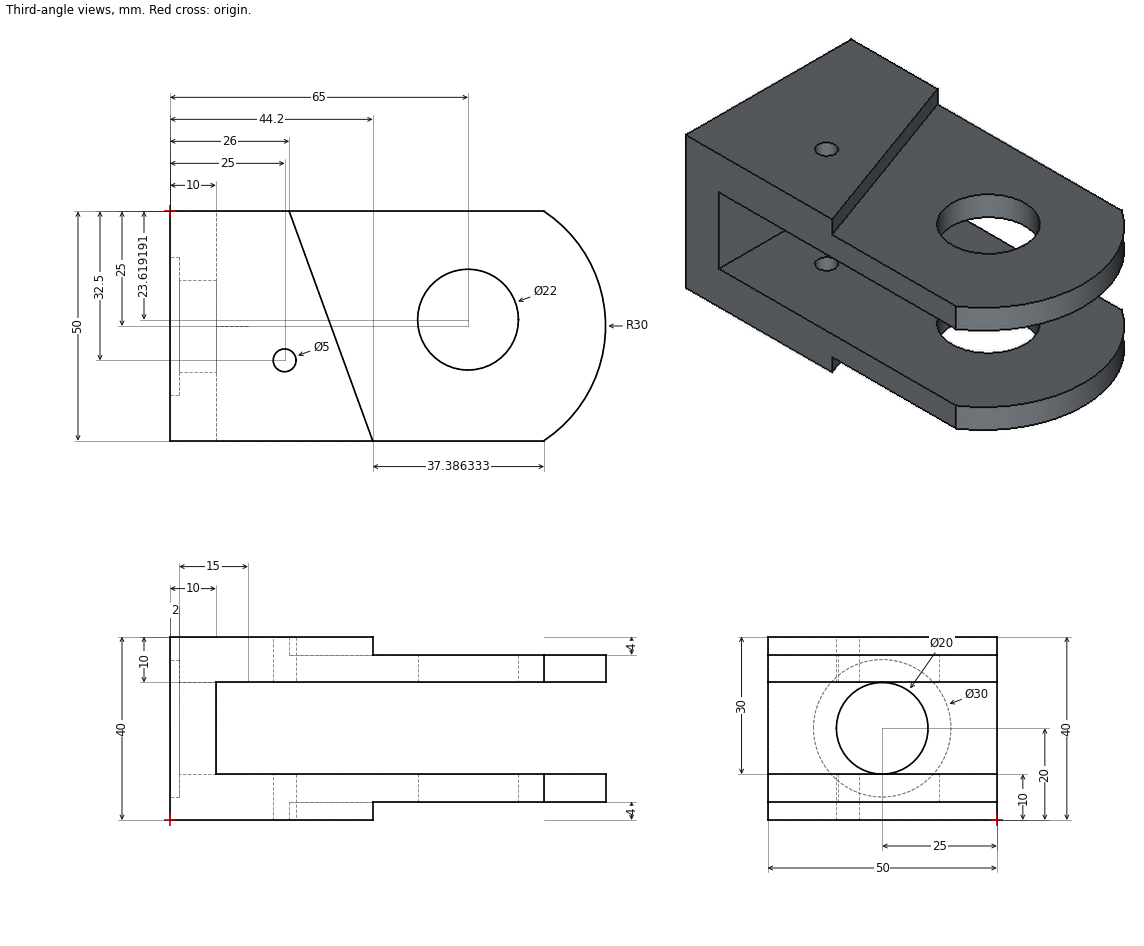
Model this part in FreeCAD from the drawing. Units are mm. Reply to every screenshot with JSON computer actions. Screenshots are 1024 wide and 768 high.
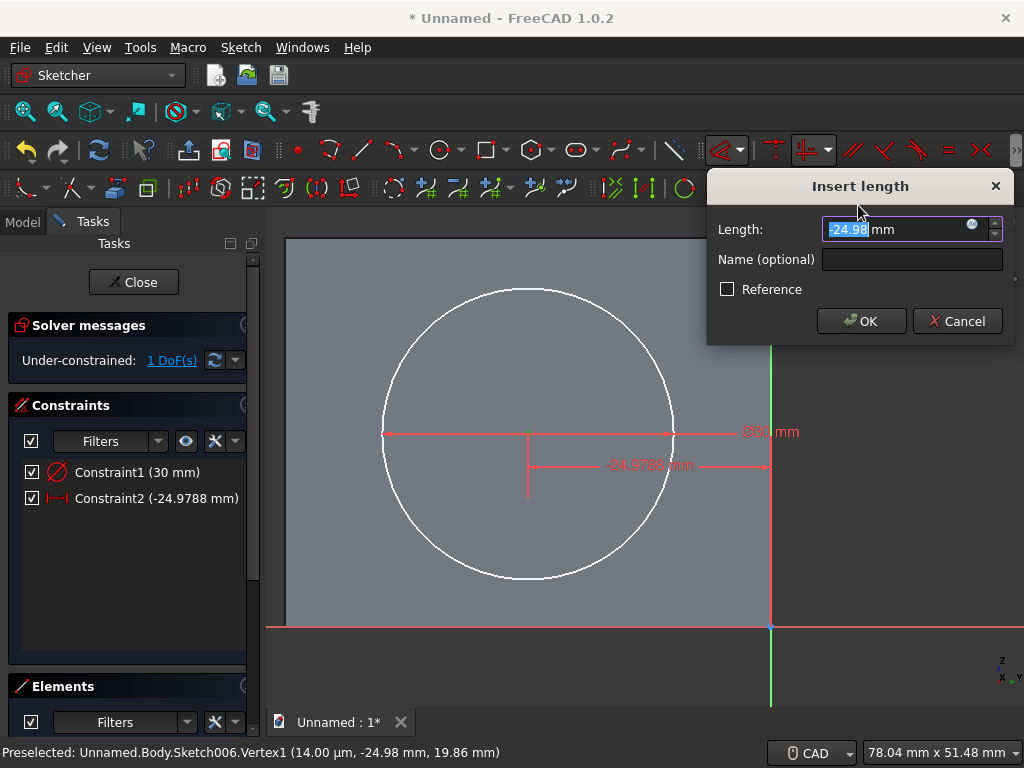
{"action": "type", "text": "-25"}
{"action": "key", "text": "Return"}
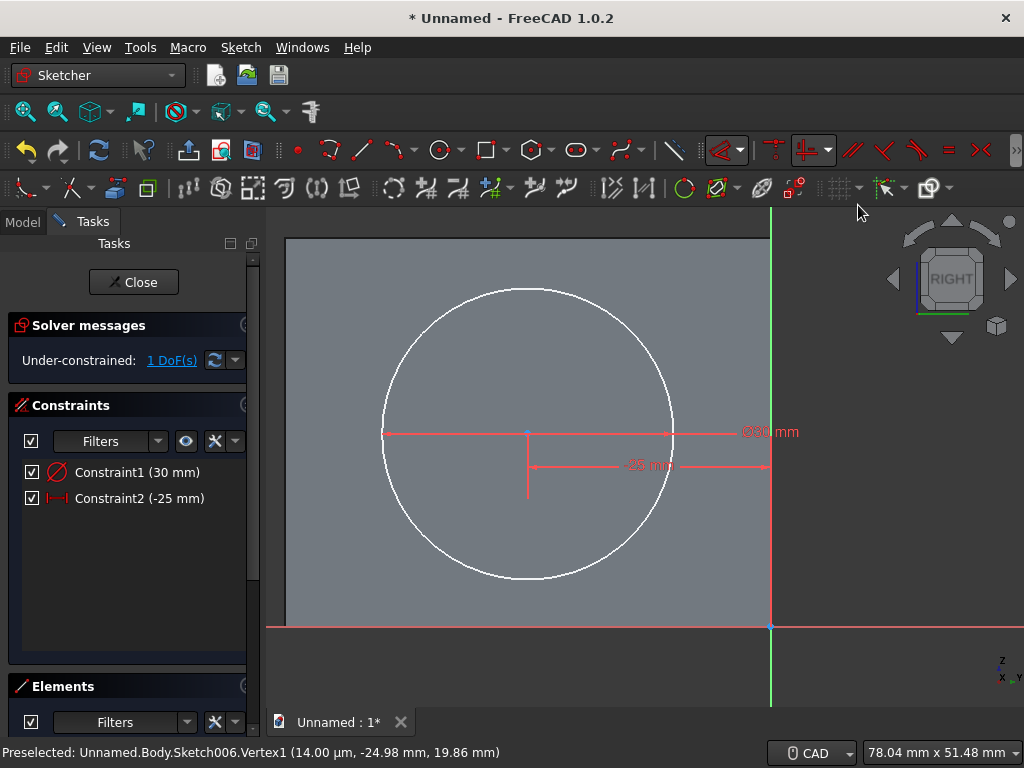
{"action": "left_click", "coordinate": [528, 434]}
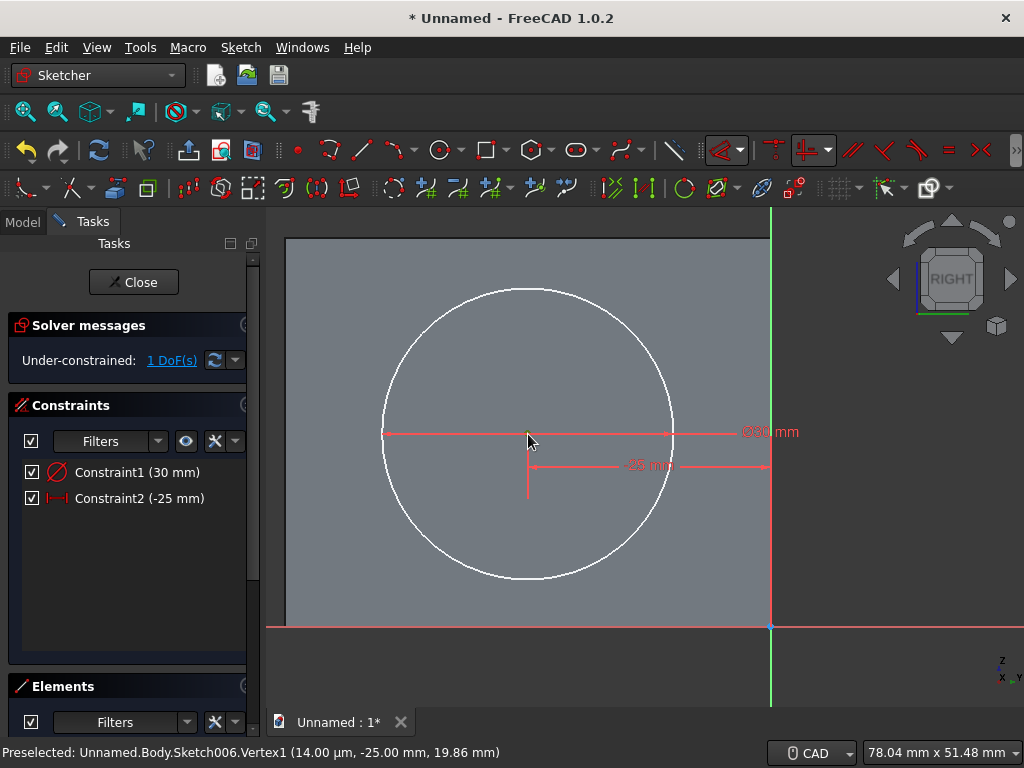
{"action": "key", "text": "i"}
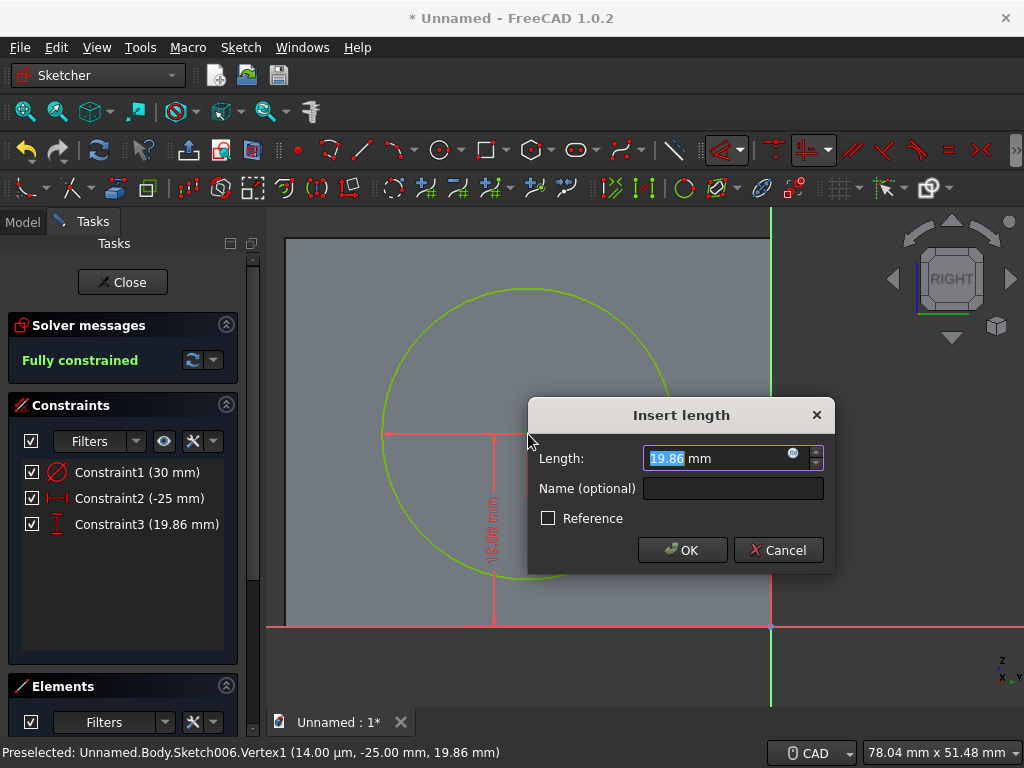
{"action": "type", "text": "20"}
{"action": "key", "text": "Return"}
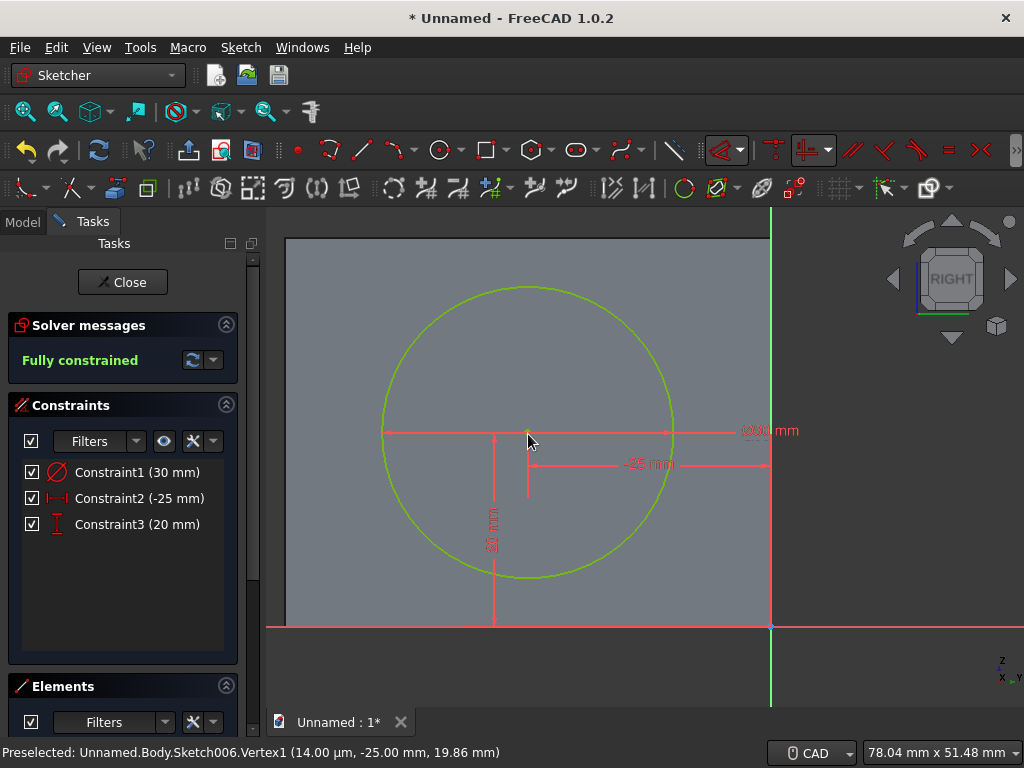
{"action": "left_click", "coordinate": [123, 282]}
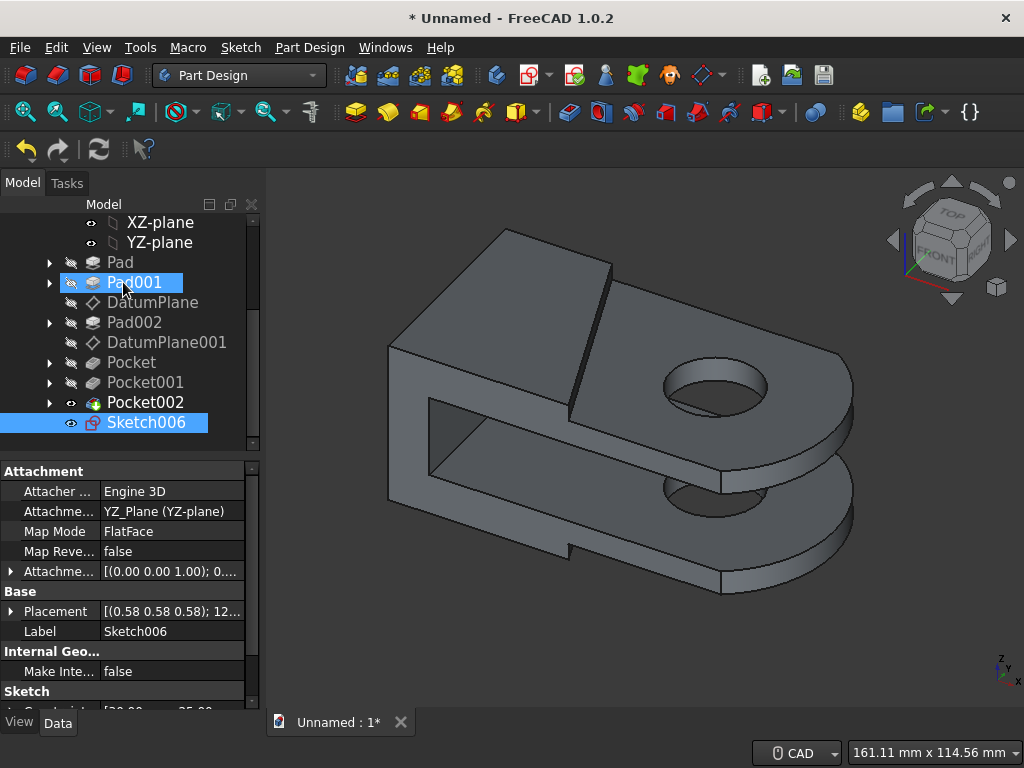
{"action": "left_click", "coordinate": [570, 112]}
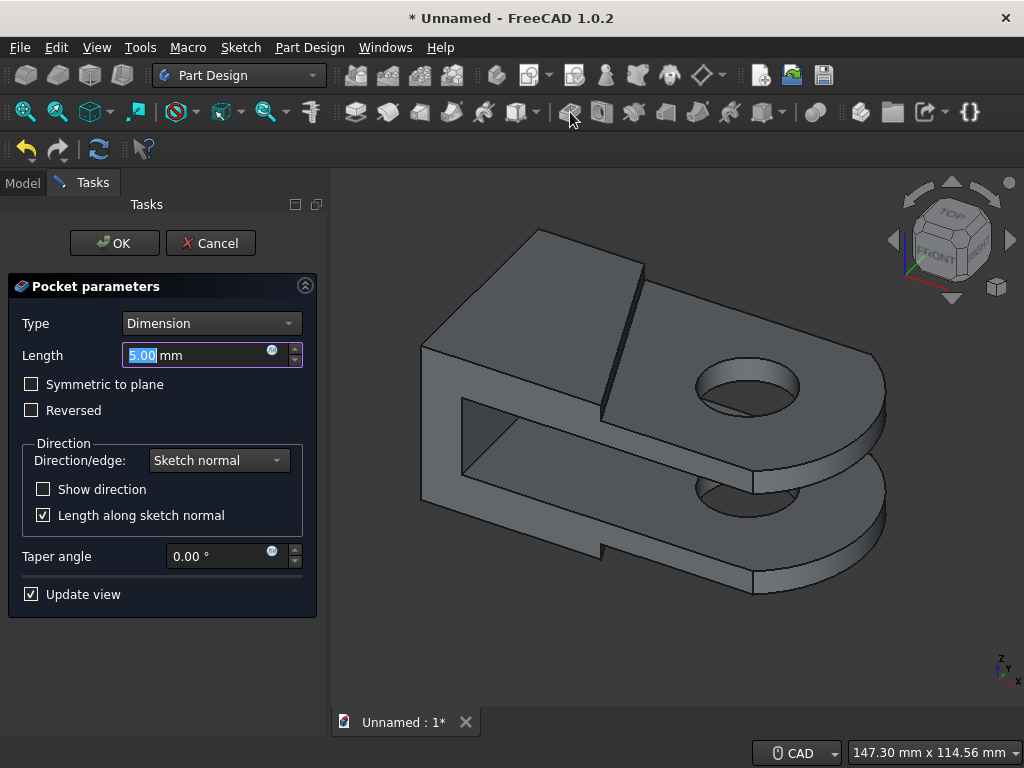
{"action": "type", "text": "2"}
{"action": "key", "text": "Tab"}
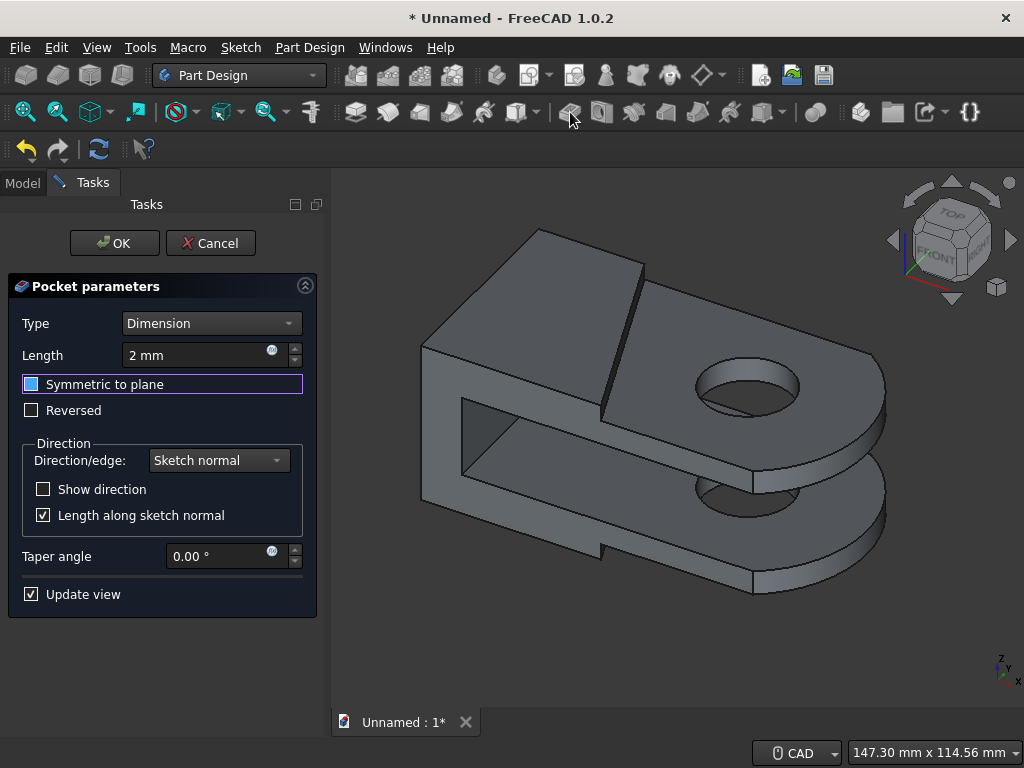
{"action": "left_click", "coordinate": [30, 410]}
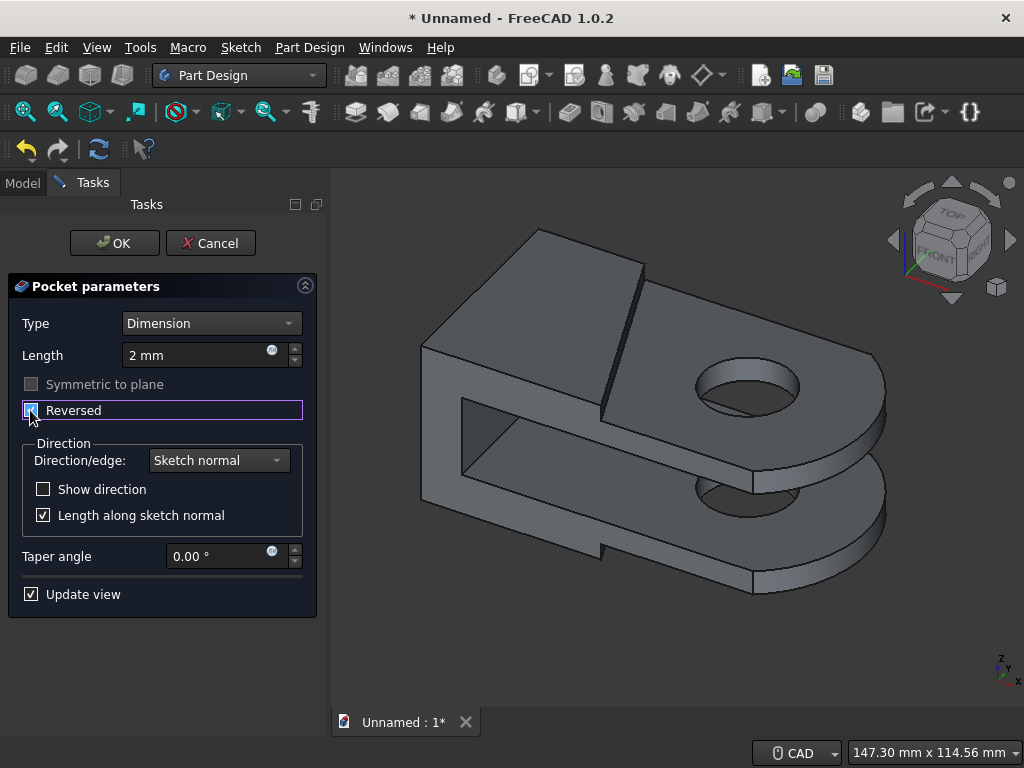
{"action": "left_click", "coordinate": [115, 243]}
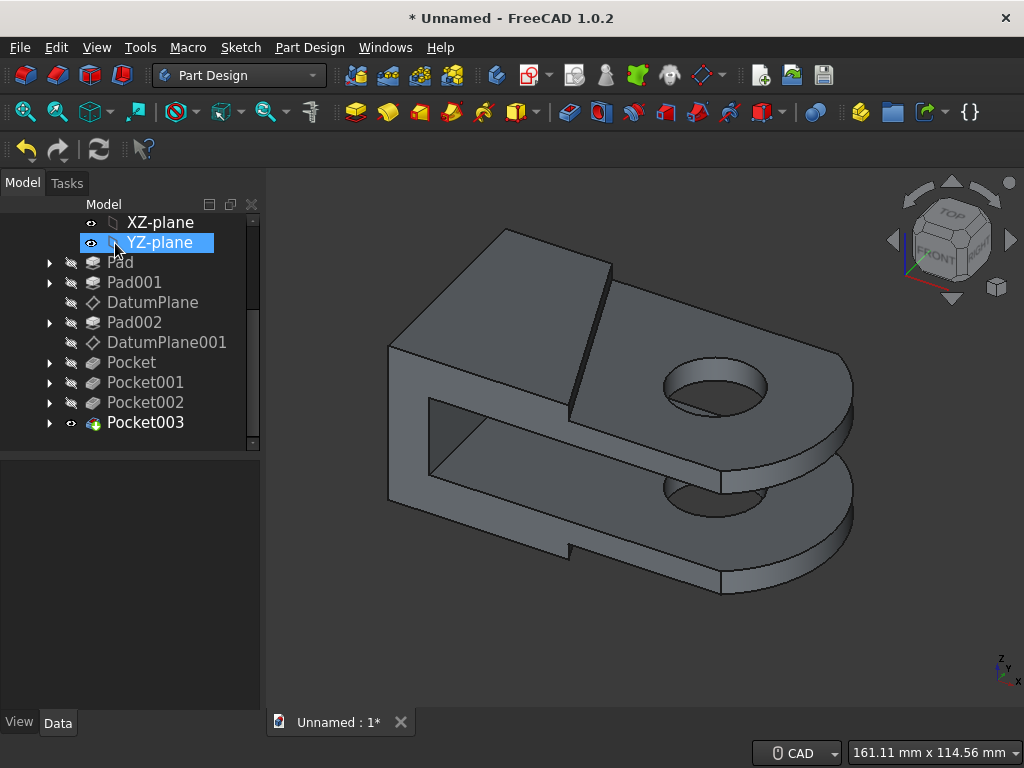
{"action": "key", "text": "6"}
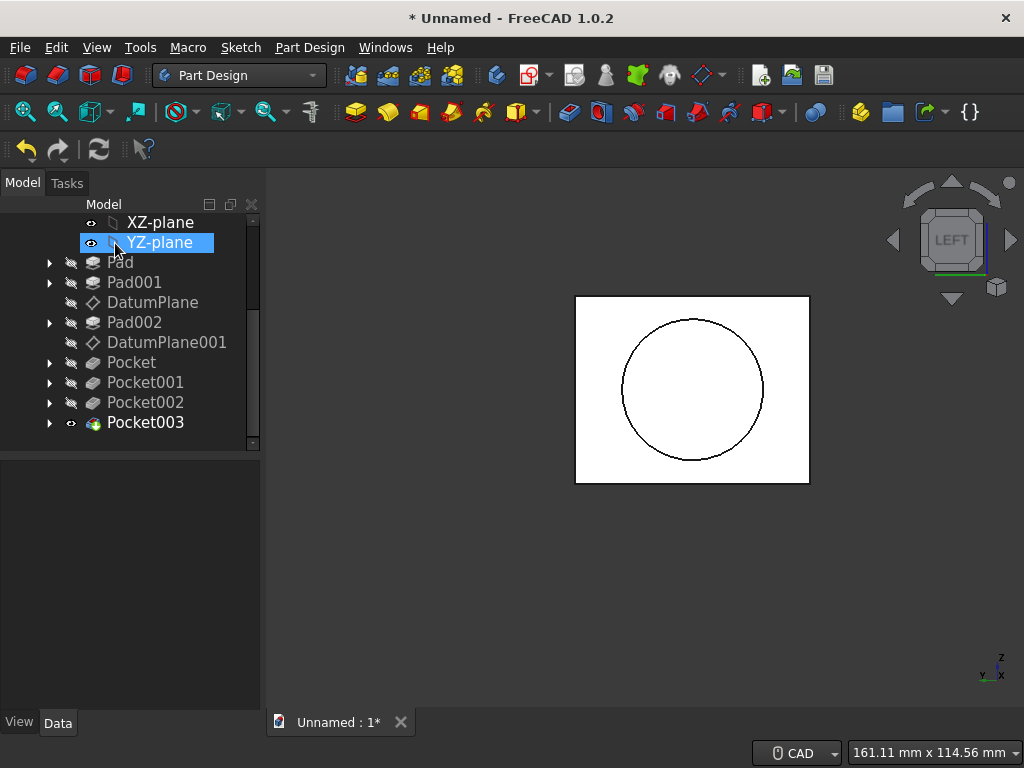
{"action": "left_click", "coordinate": [26, 112]}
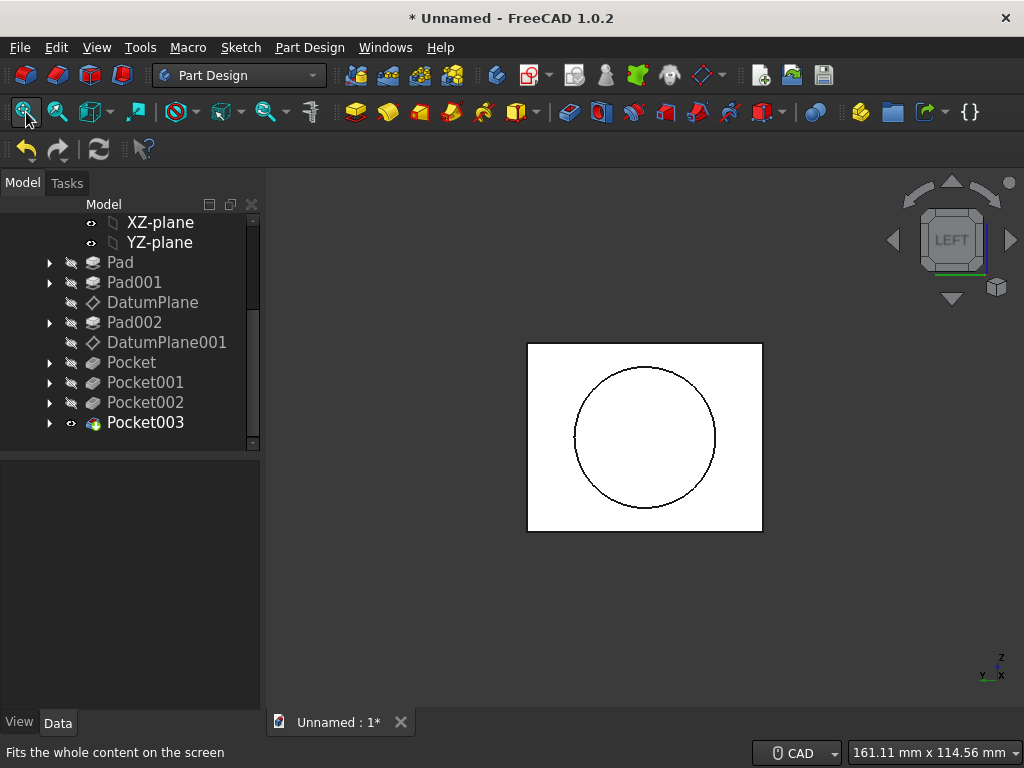
{"action": "left_click", "coordinate": [645, 436]}